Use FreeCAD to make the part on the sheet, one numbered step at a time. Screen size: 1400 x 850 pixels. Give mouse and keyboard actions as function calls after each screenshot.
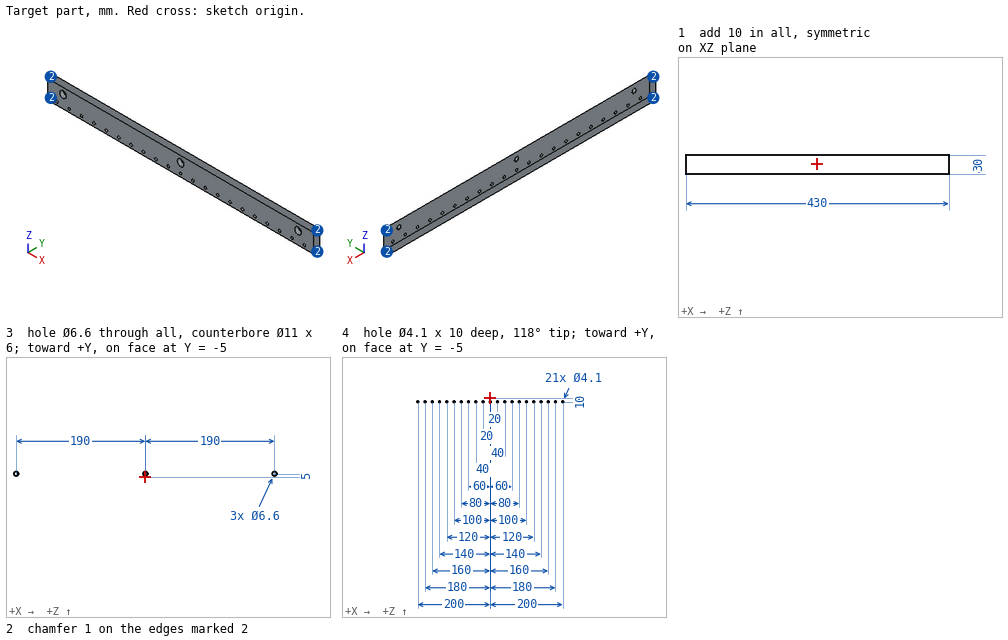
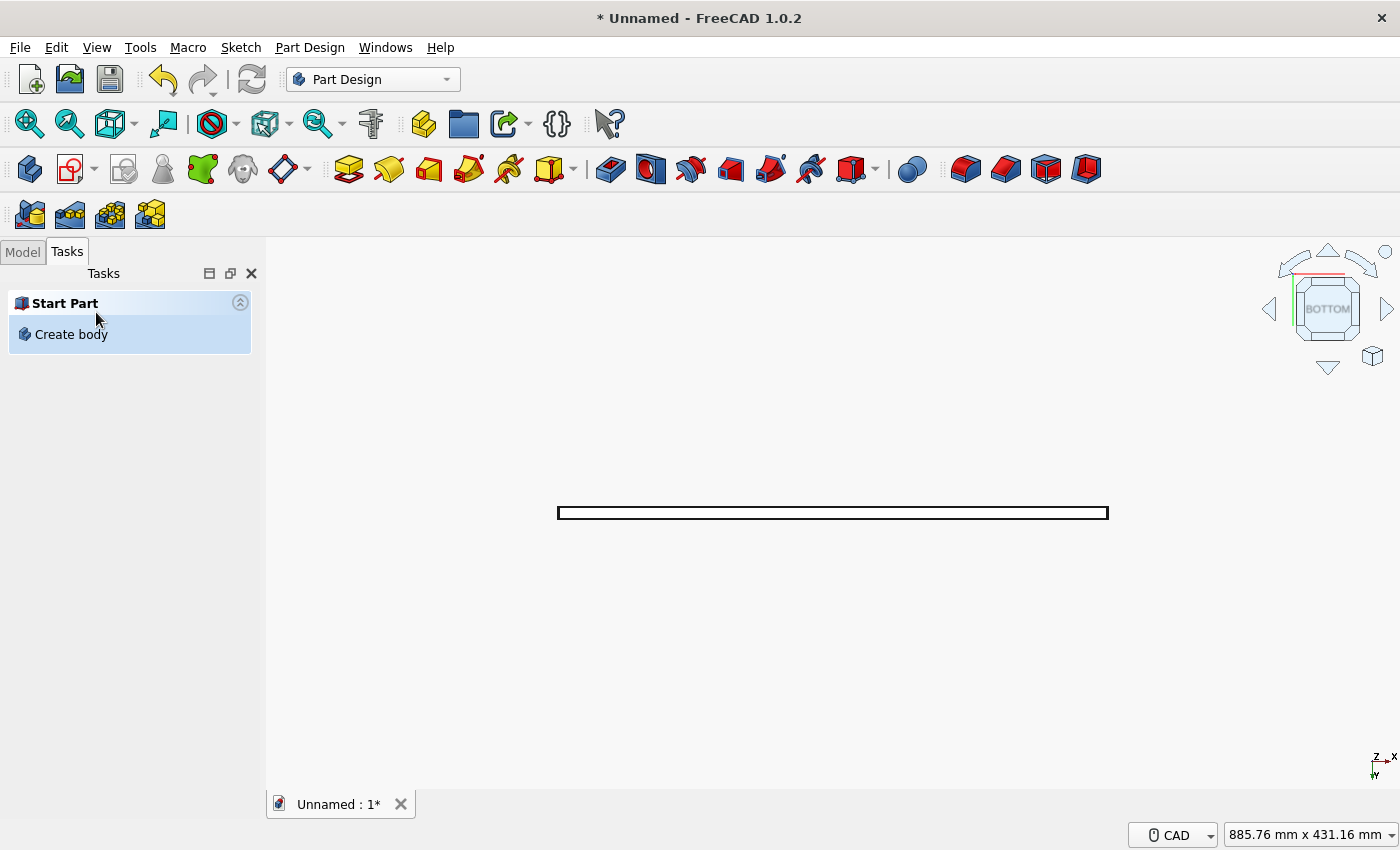
key(0)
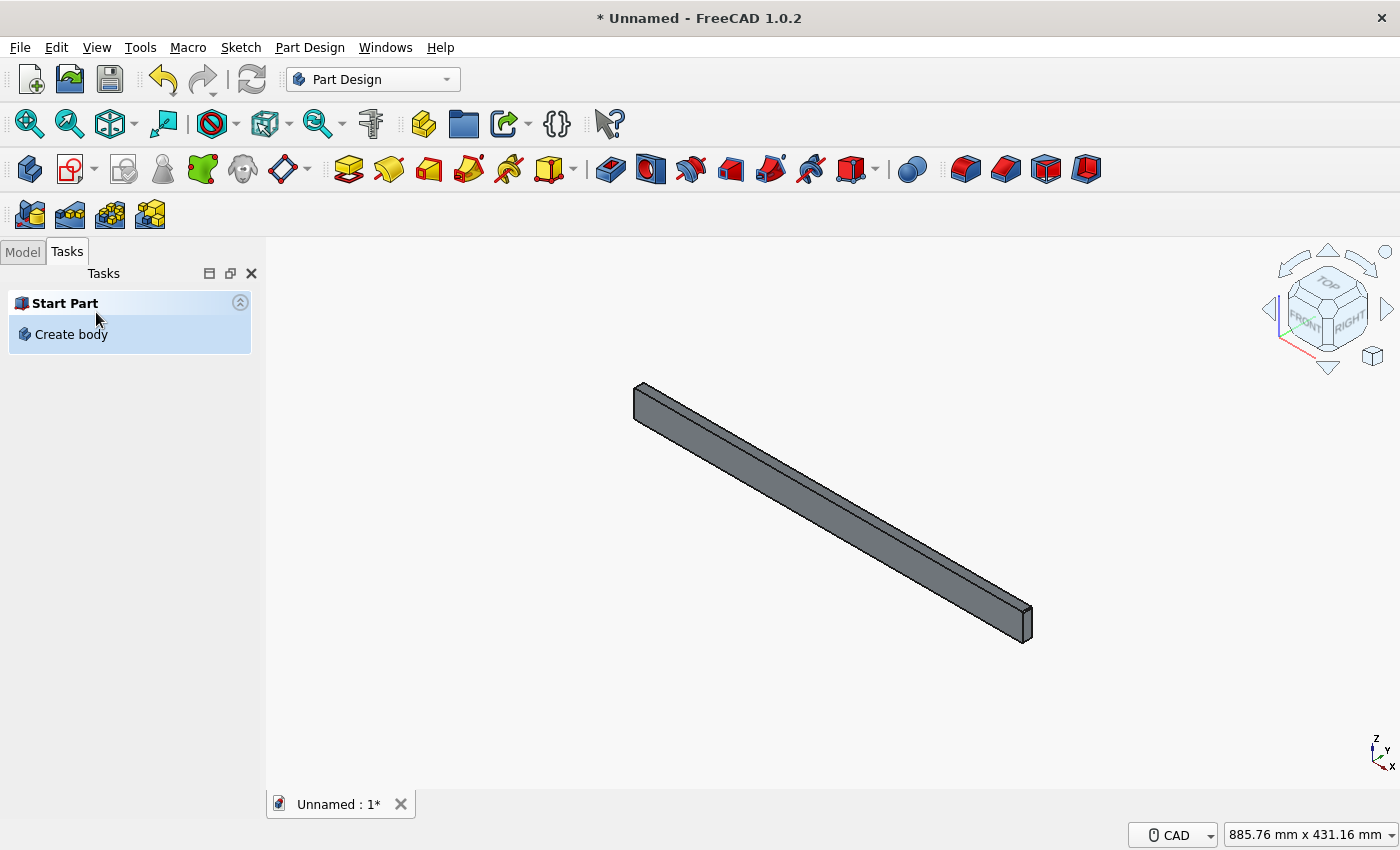
click(995, 611)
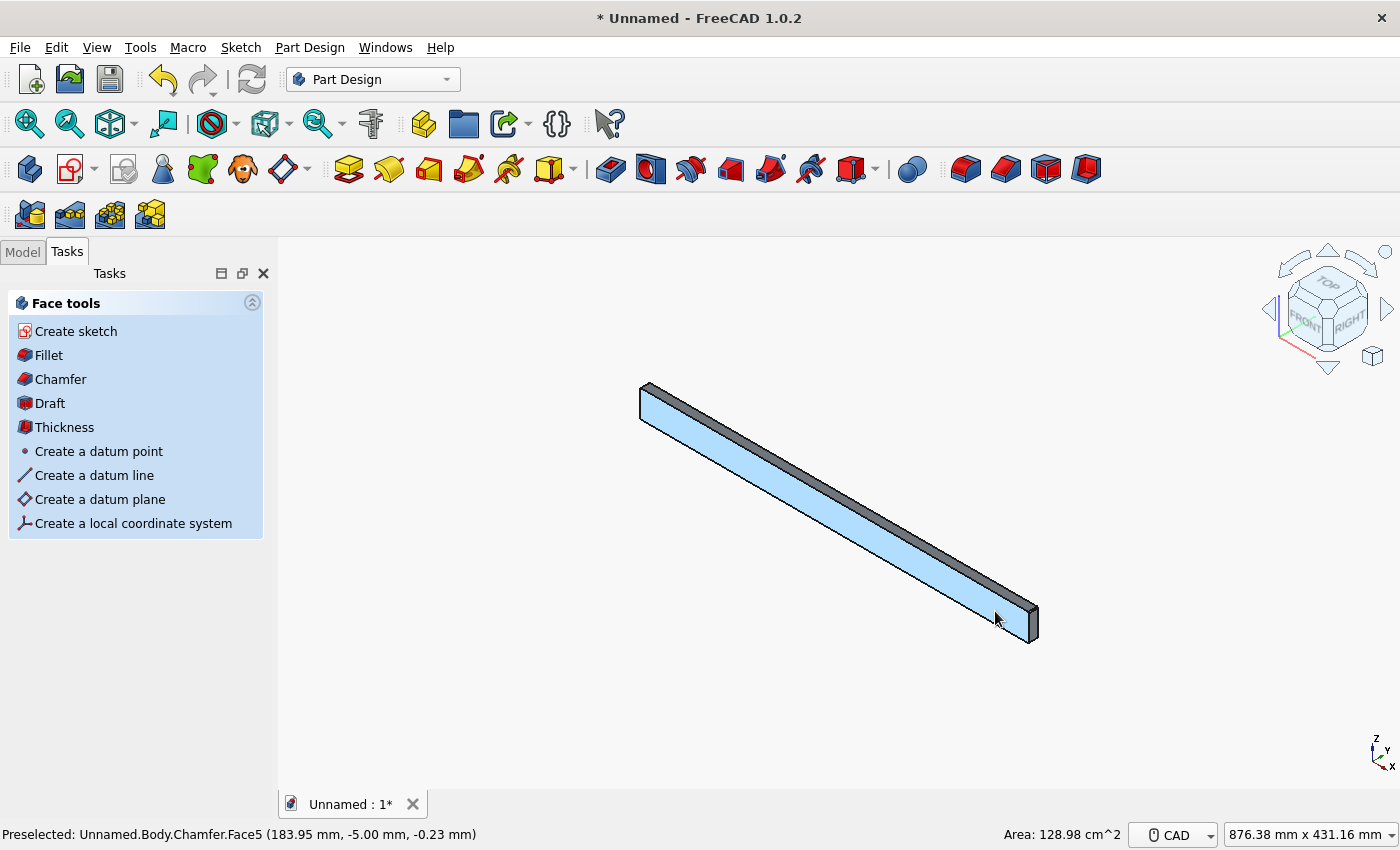
click(70, 170)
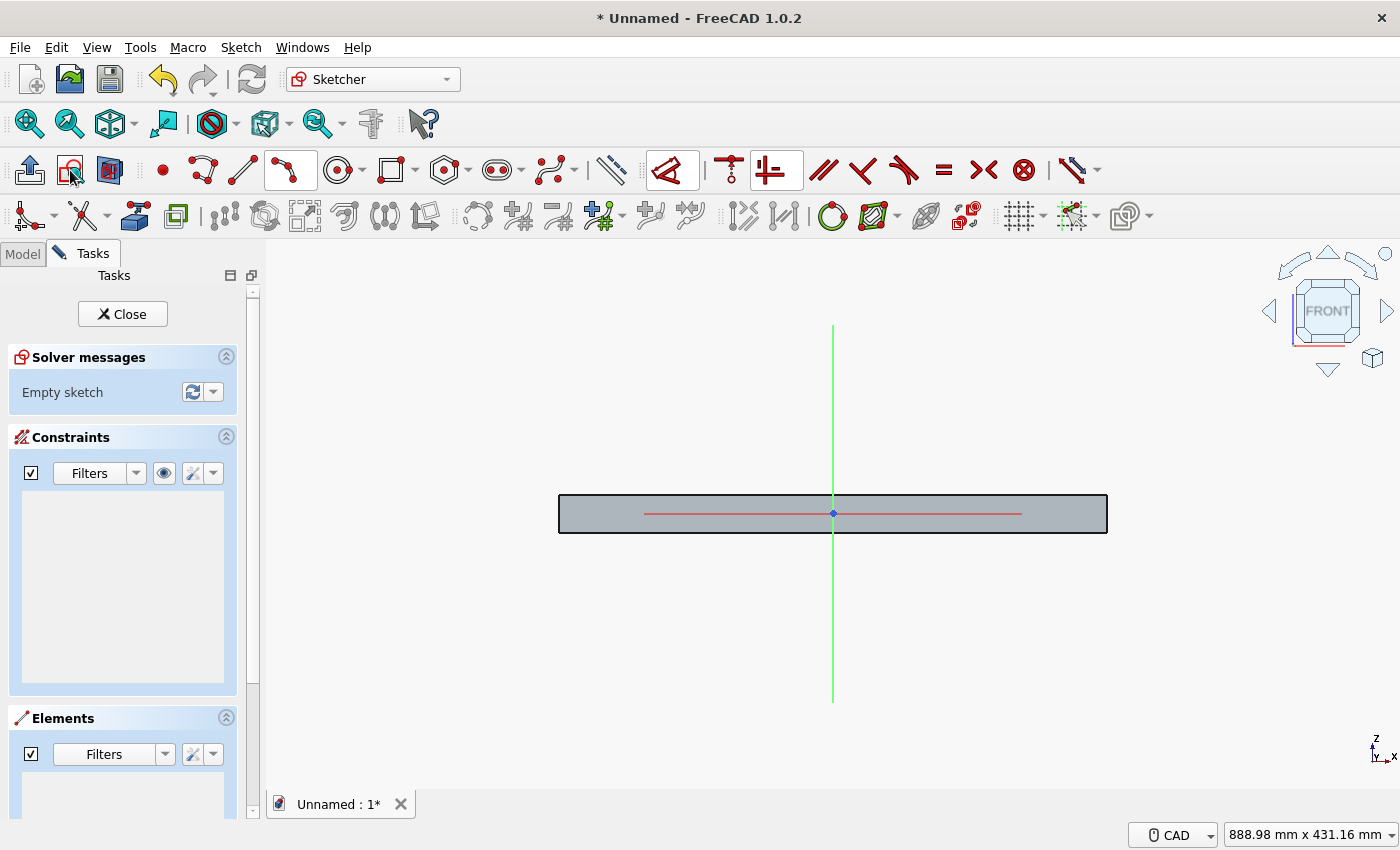
key(g)
key(c)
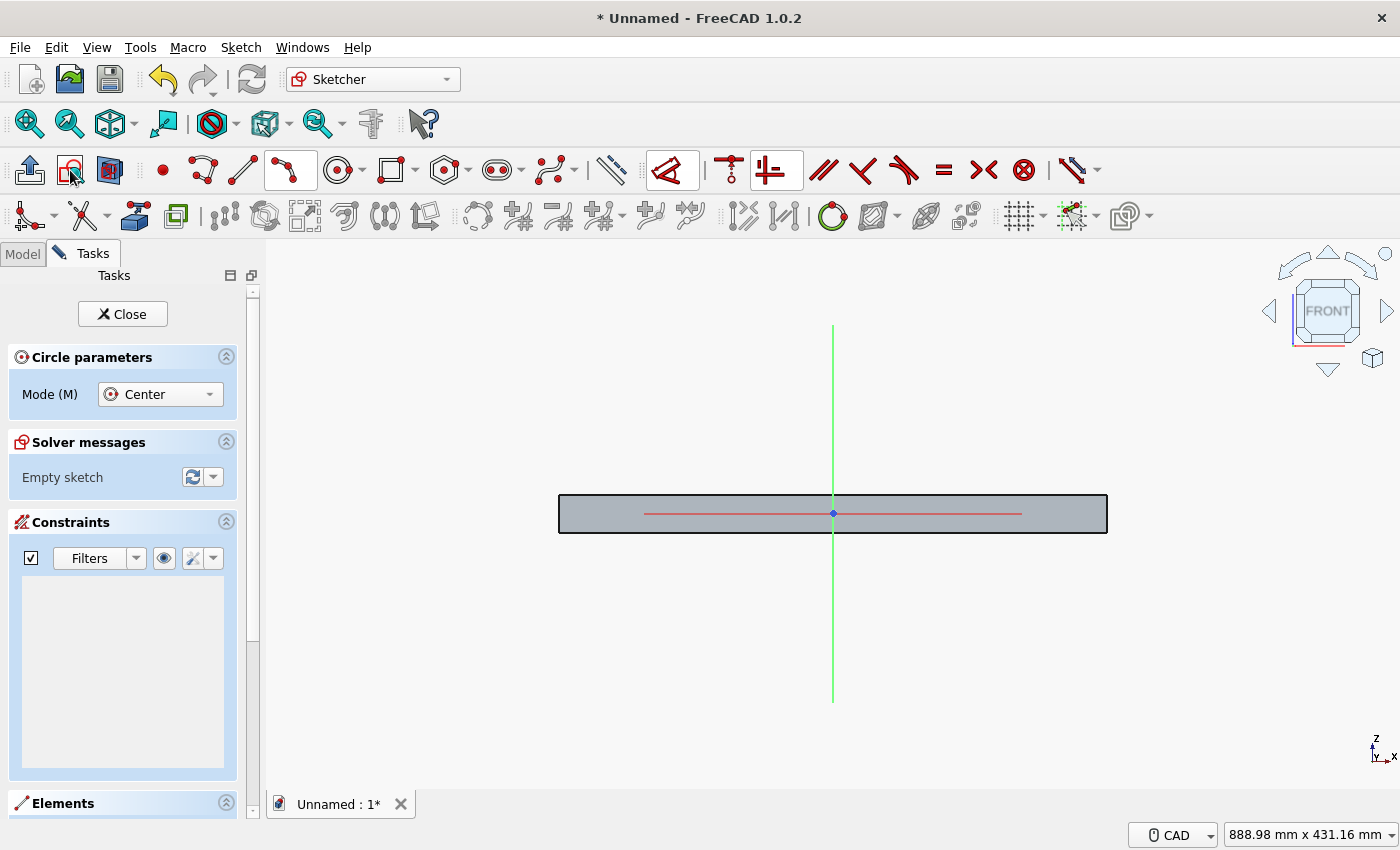
scroll(1075, 508, up, 9)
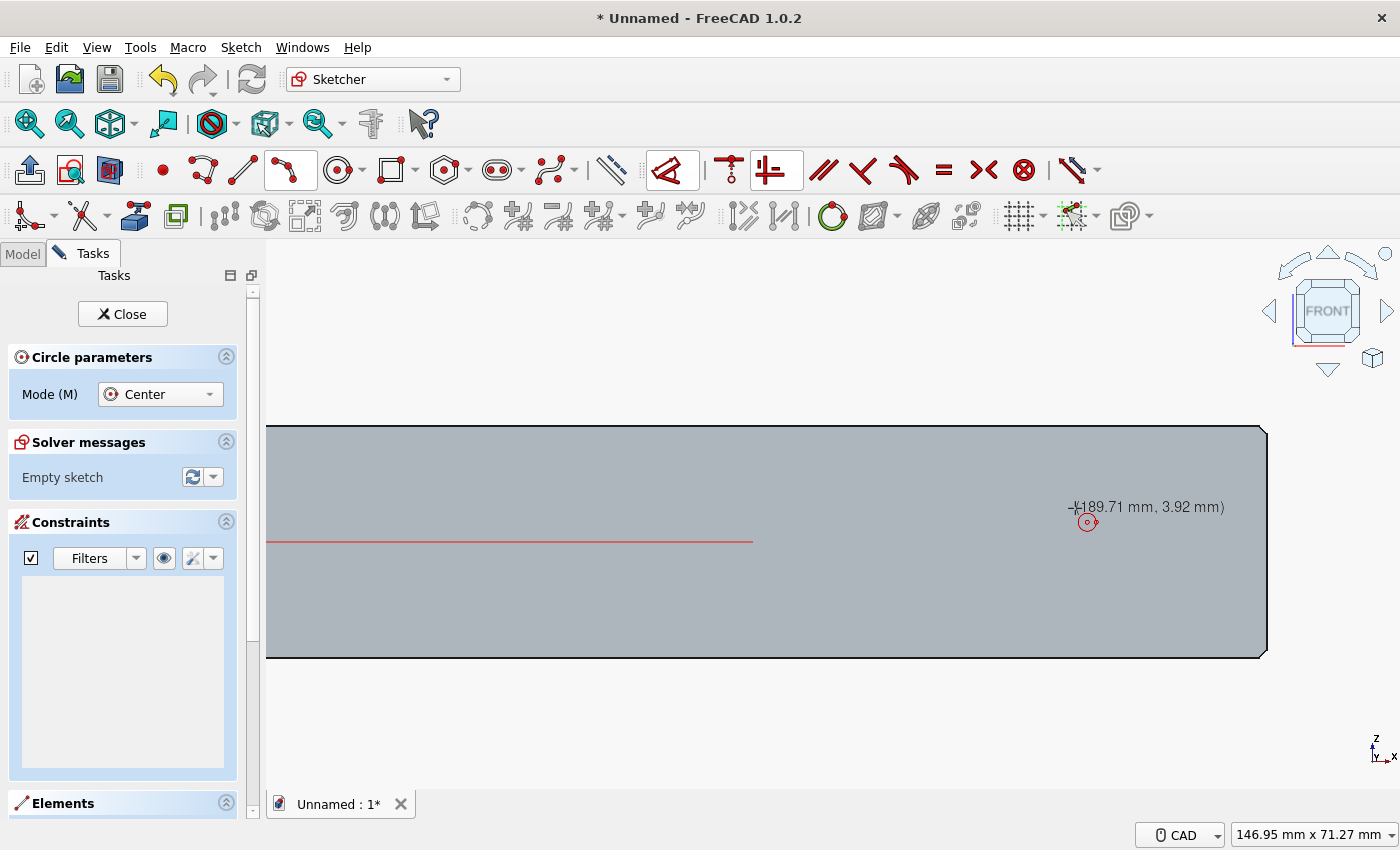
click(1074, 503)
click(1092, 485)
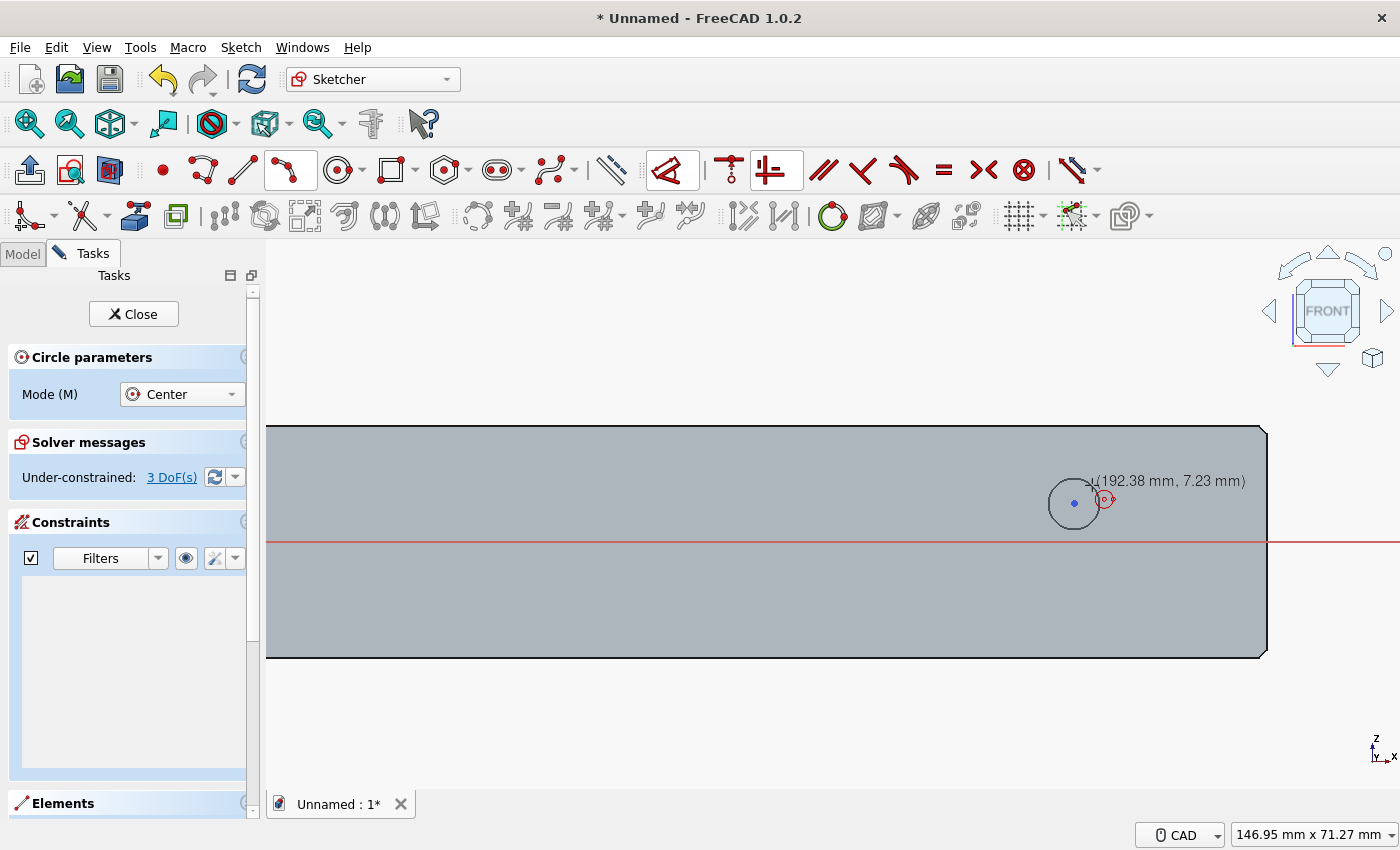
scroll(1057, 515, down, 8)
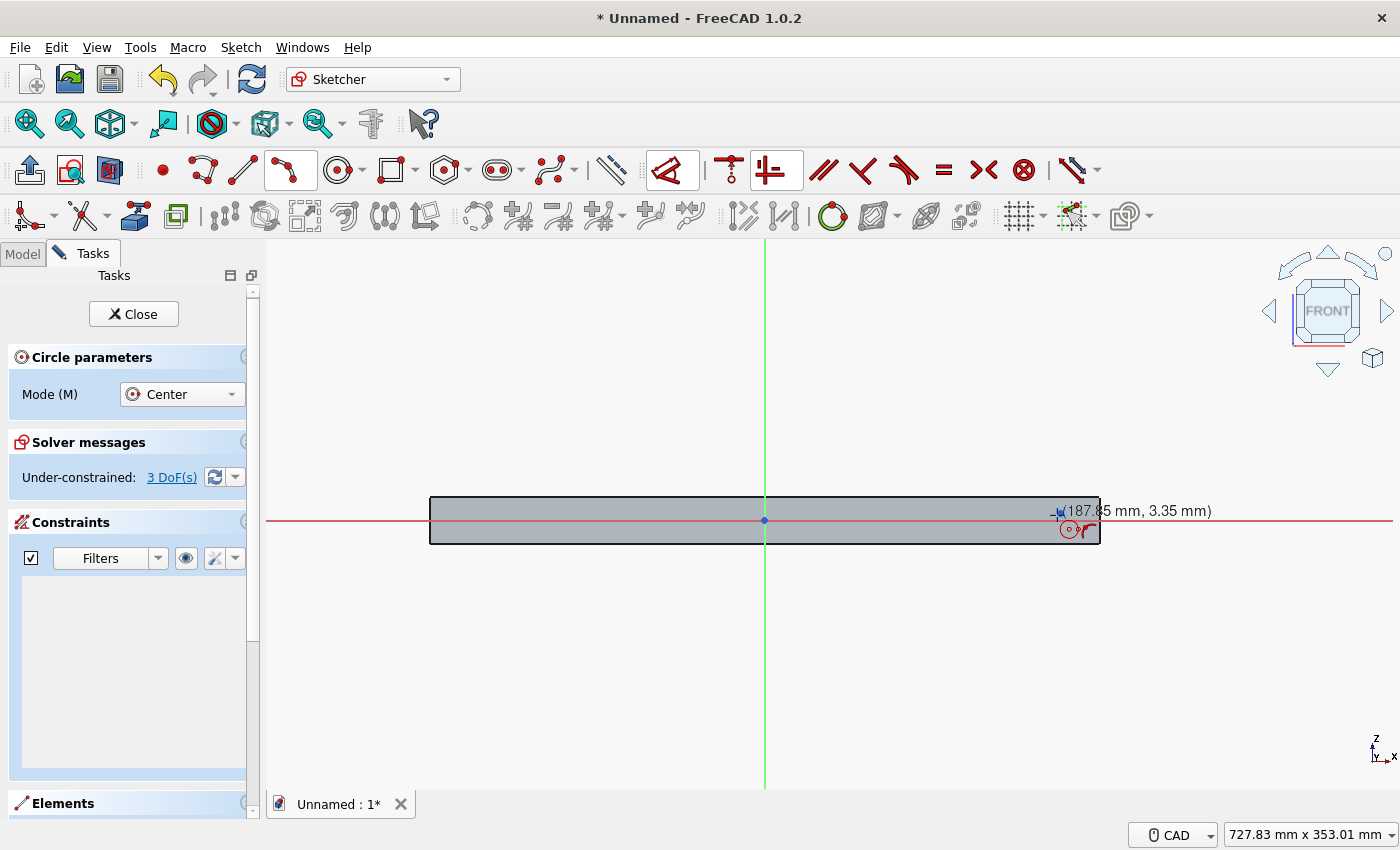
scroll(765, 513, up, 8)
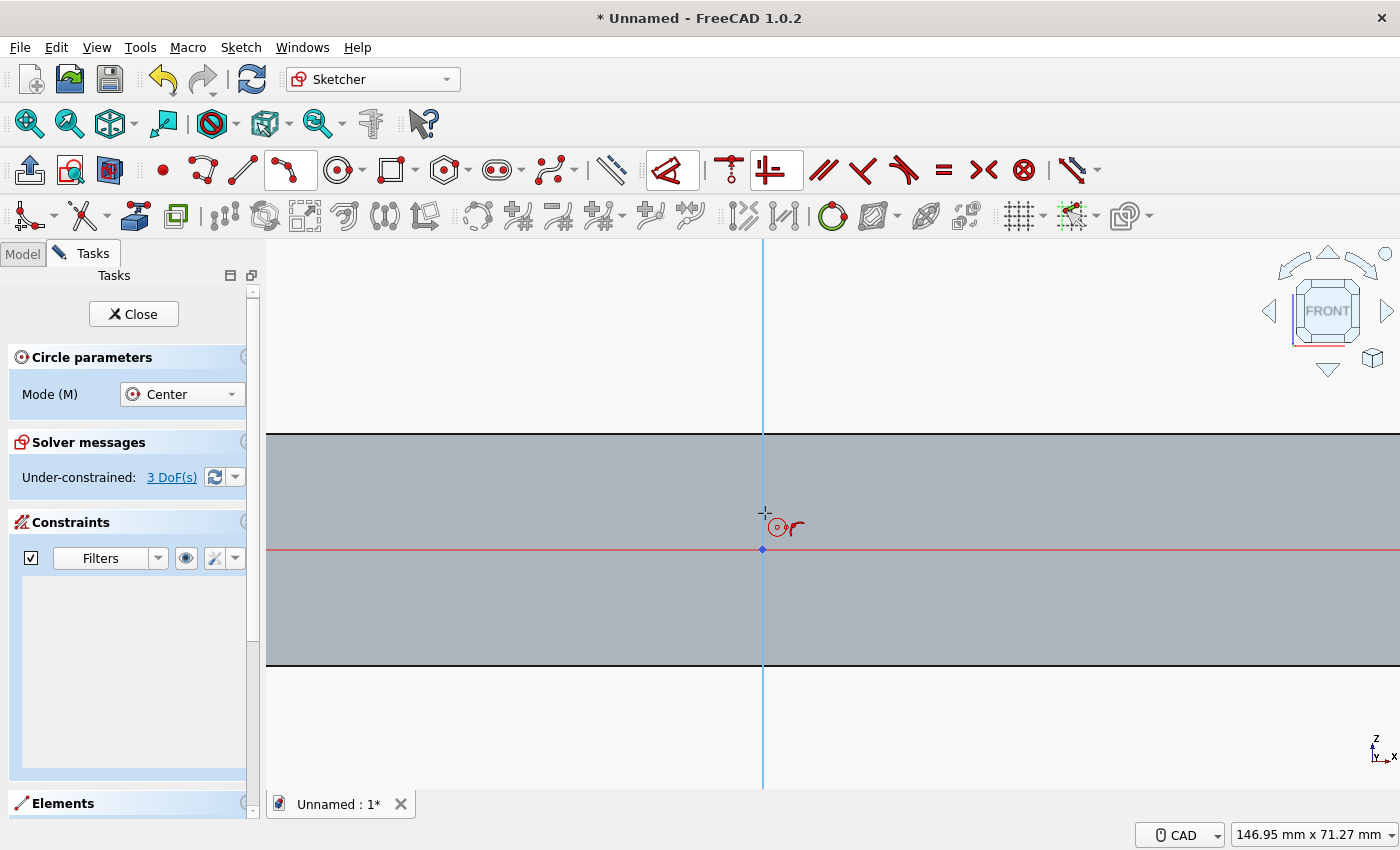
click(763, 511)
click(781, 493)